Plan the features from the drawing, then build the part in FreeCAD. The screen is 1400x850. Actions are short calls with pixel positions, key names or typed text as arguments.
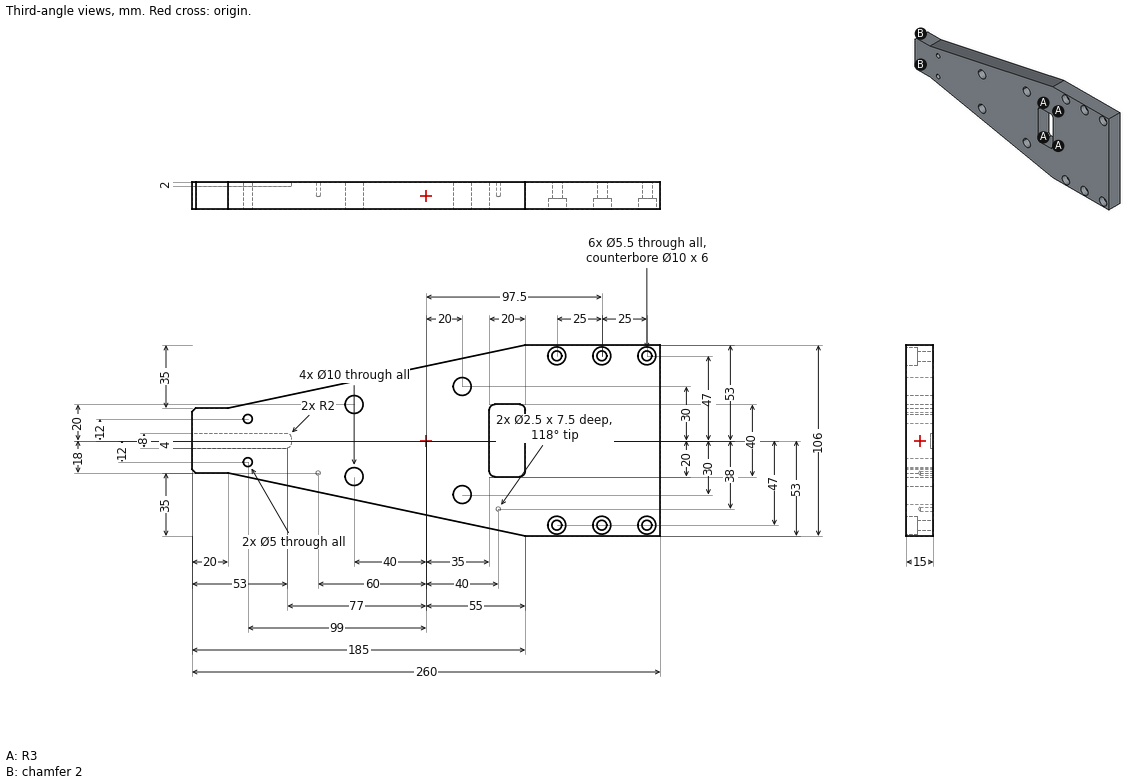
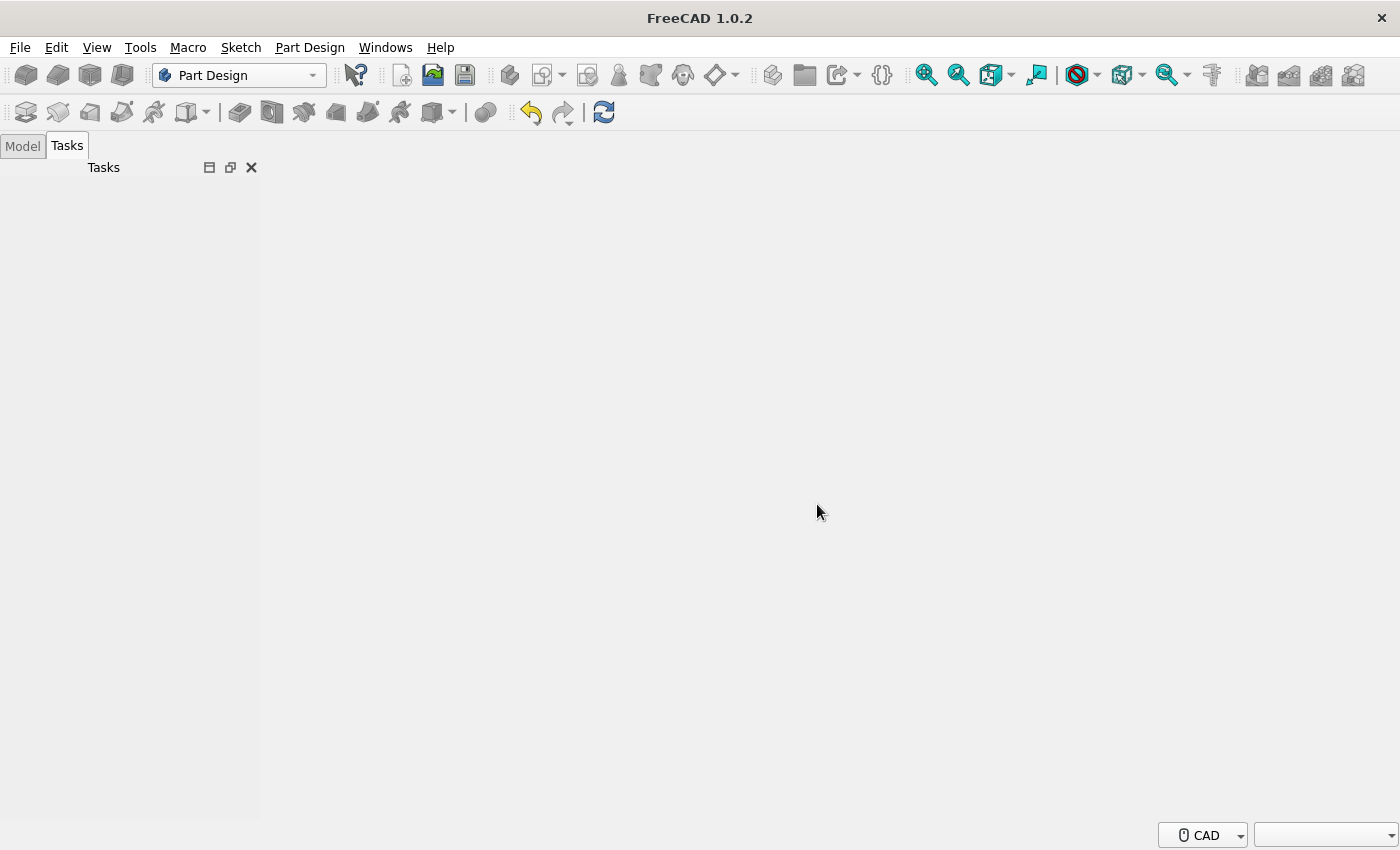
key(ctrl+n)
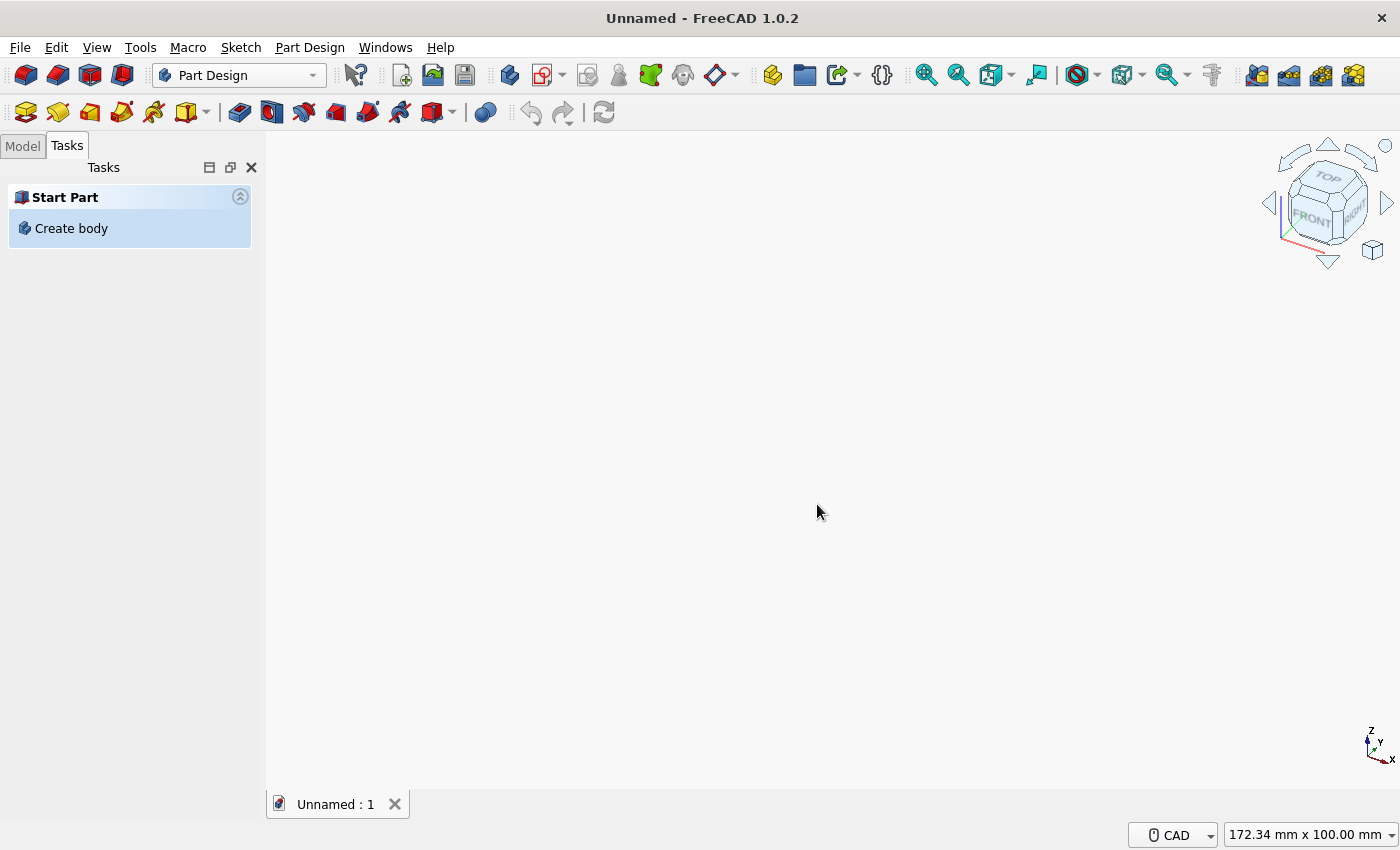
click(542, 76)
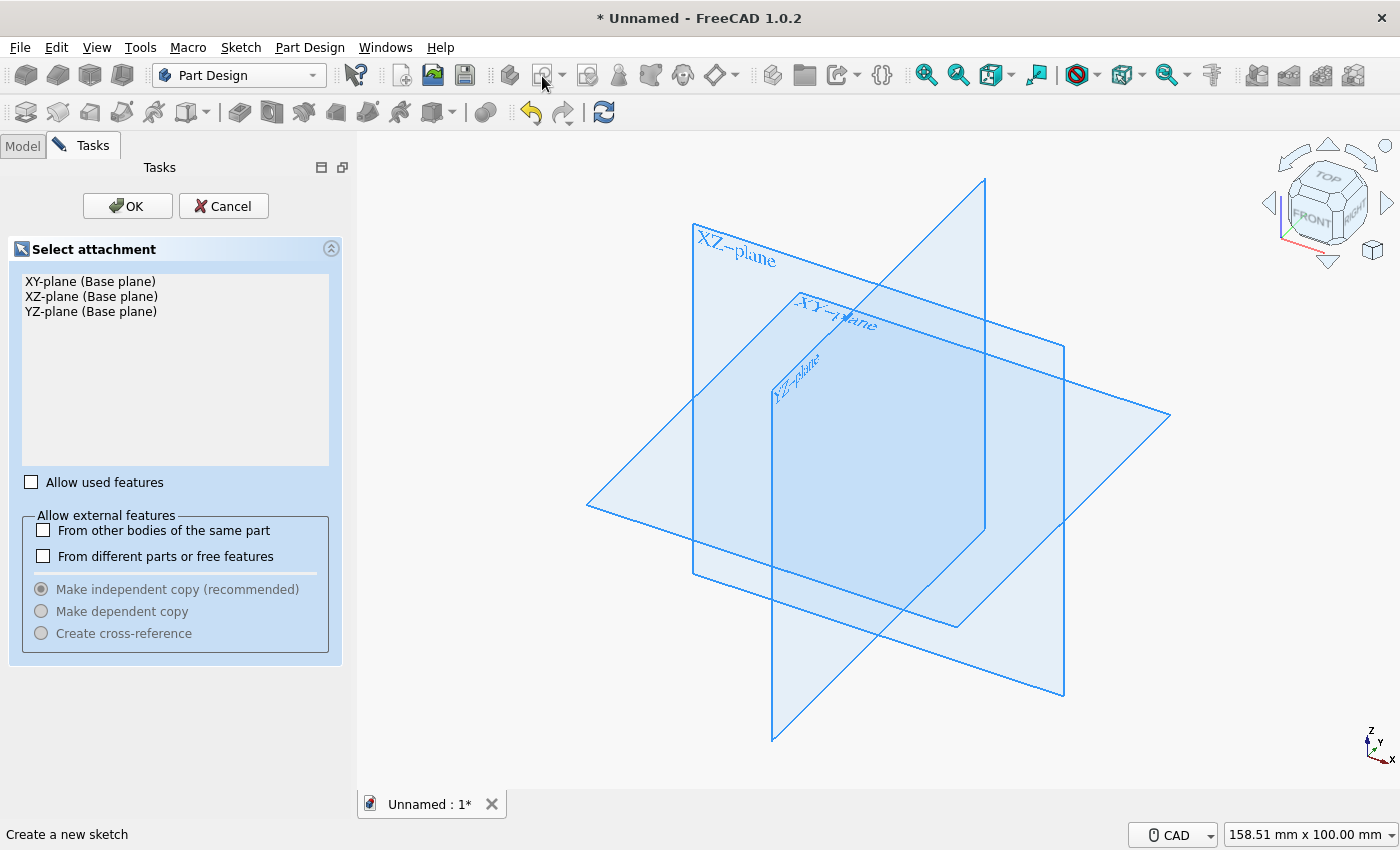
click(82, 296)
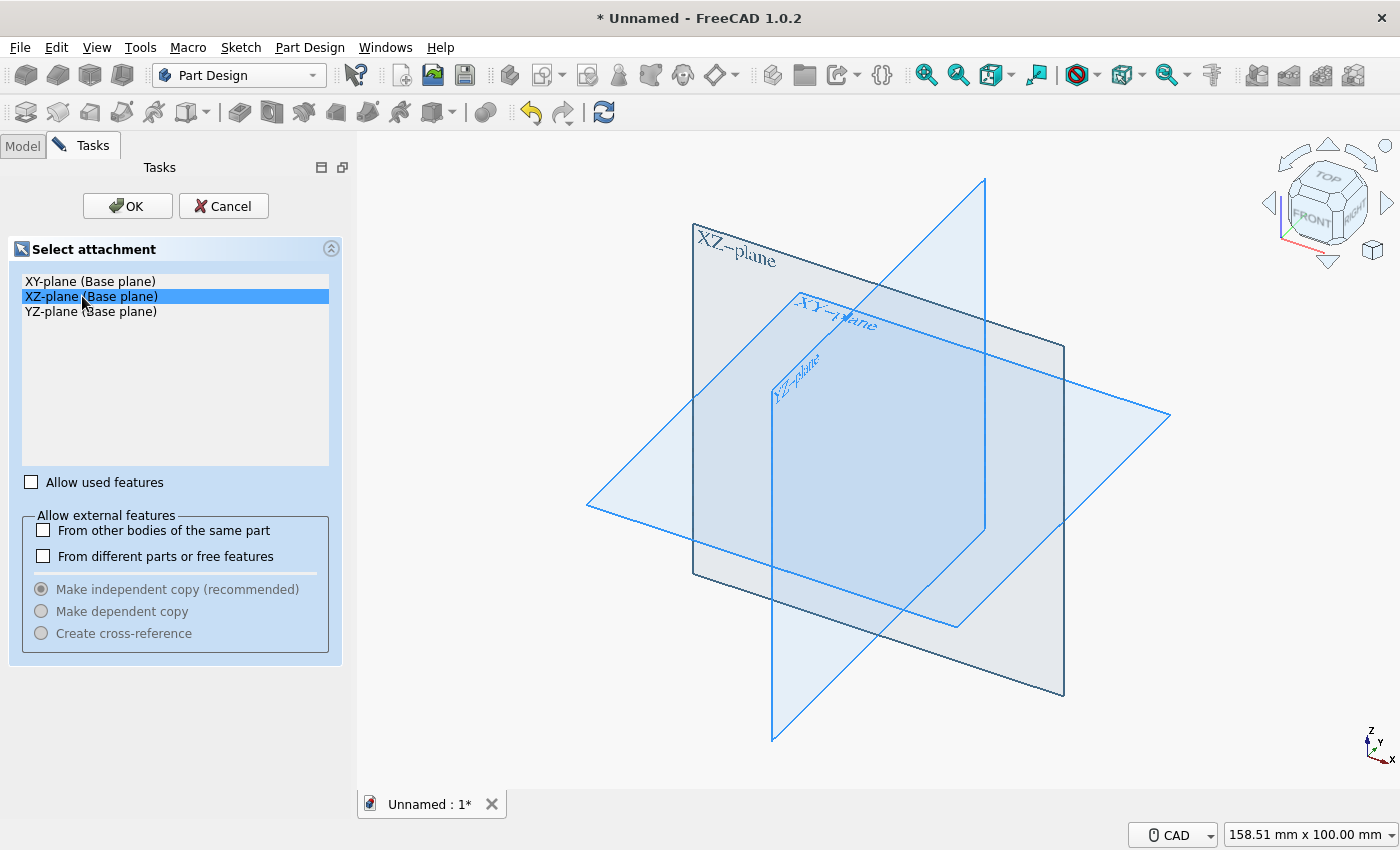
click(128, 206)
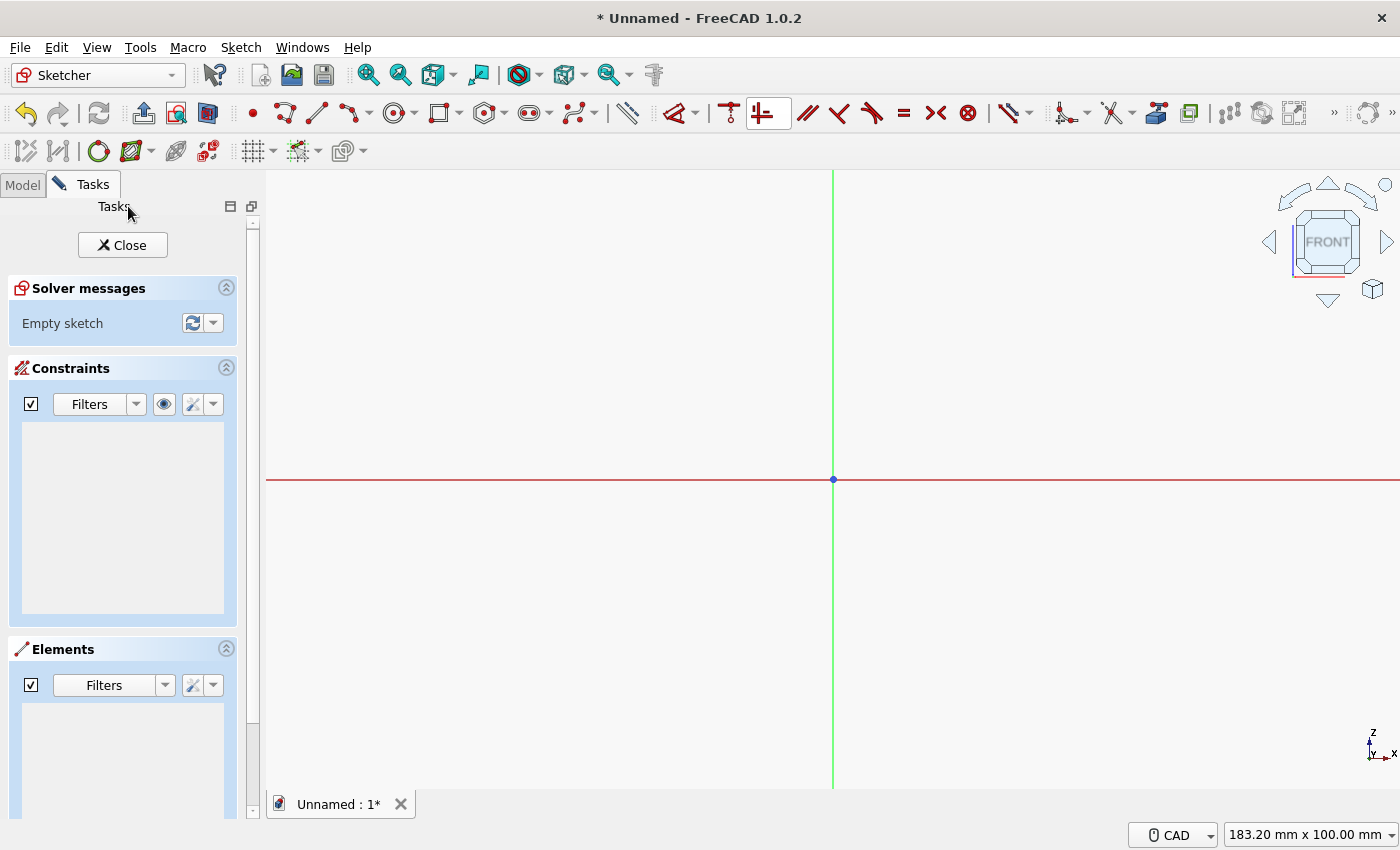
scroll(709, 480, down, 4)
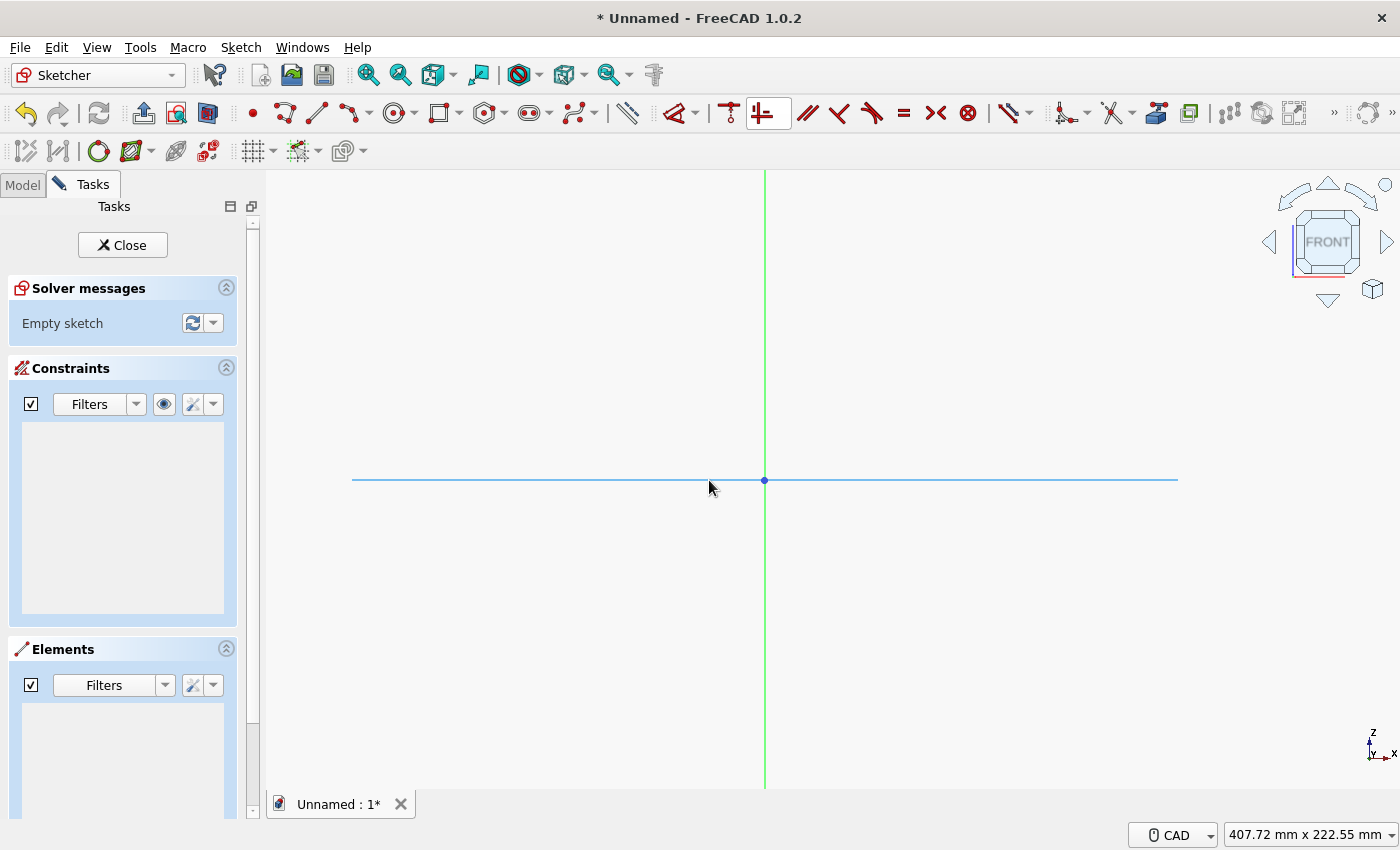
key(g)
key(v)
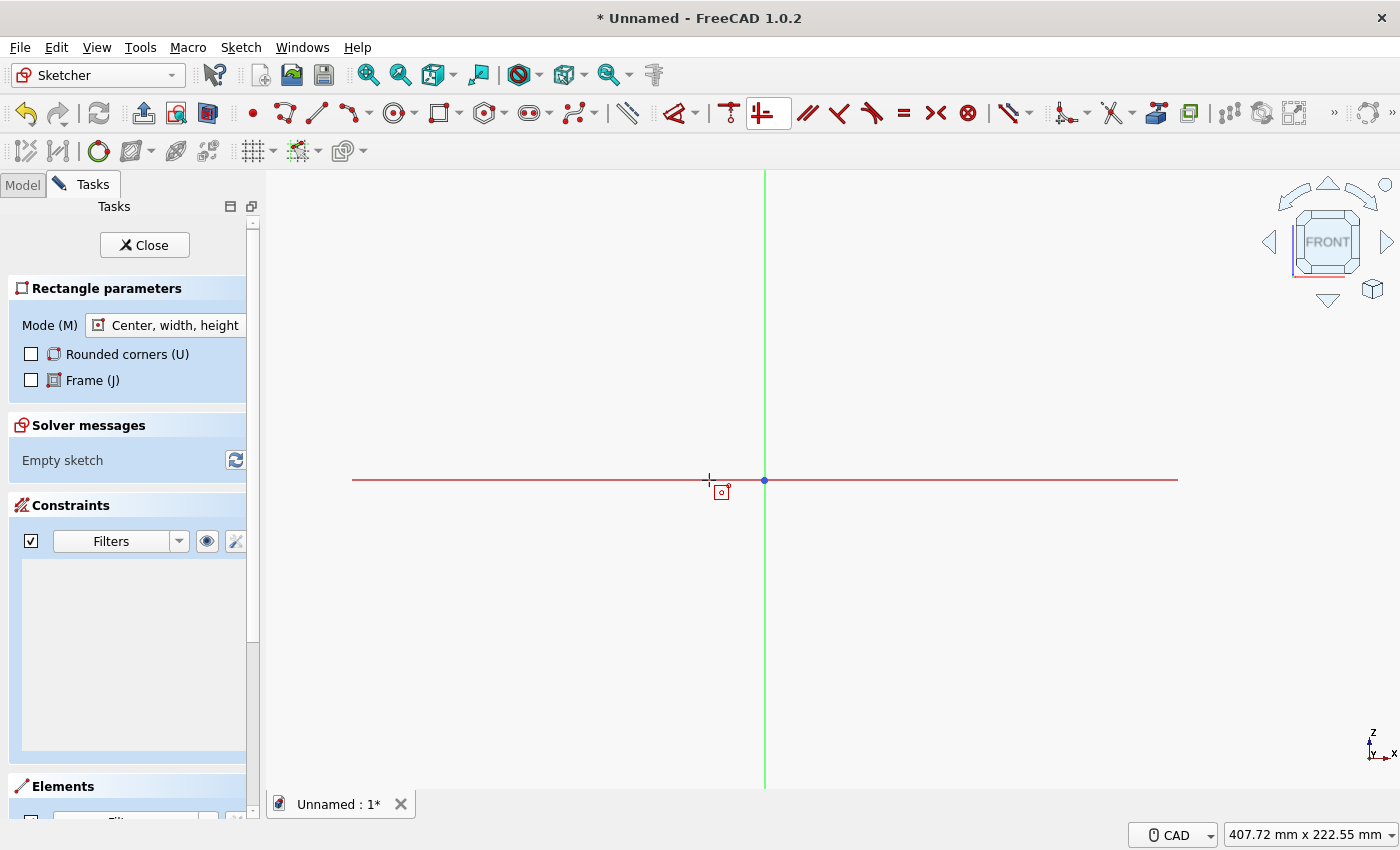
click(765, 480)
click(1127, 333)
key(Escape)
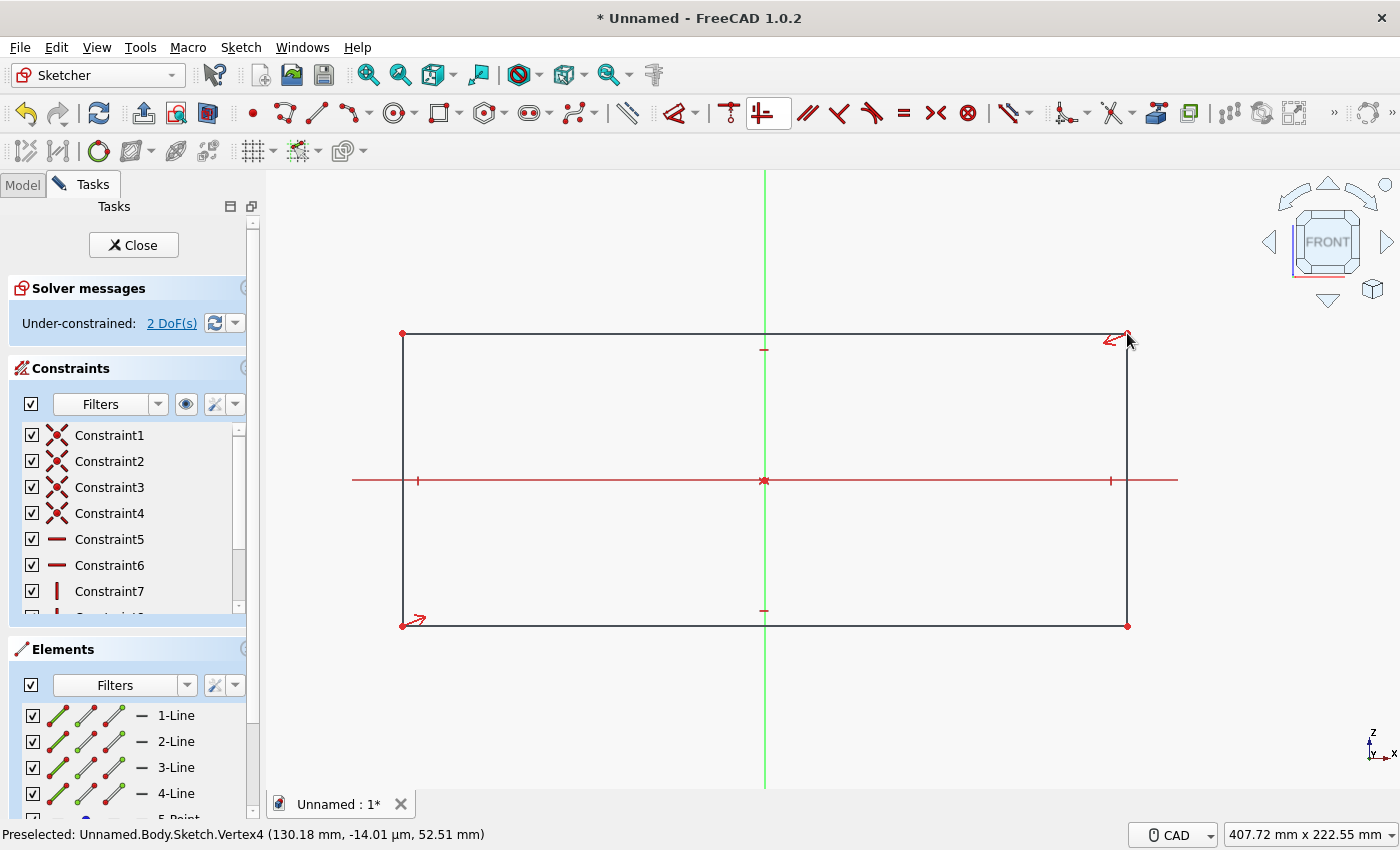
key(d)